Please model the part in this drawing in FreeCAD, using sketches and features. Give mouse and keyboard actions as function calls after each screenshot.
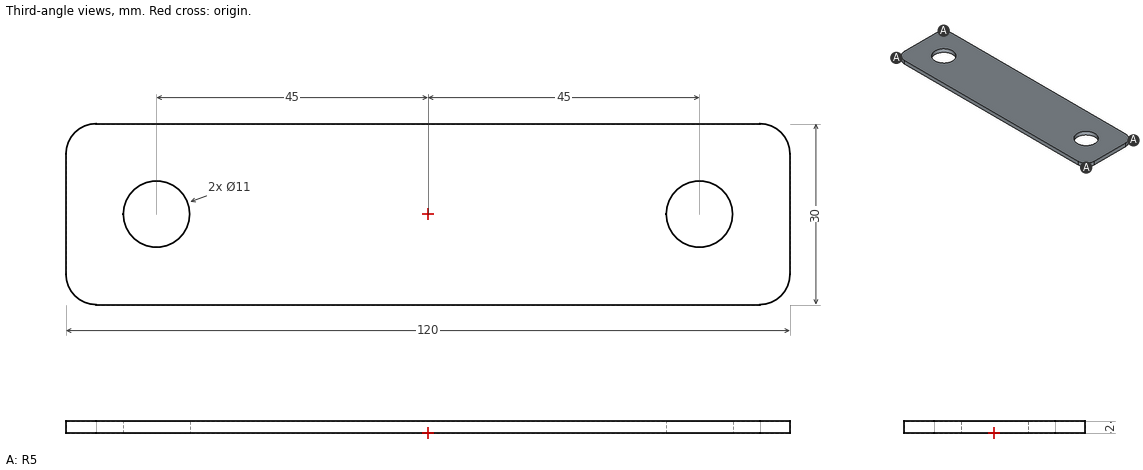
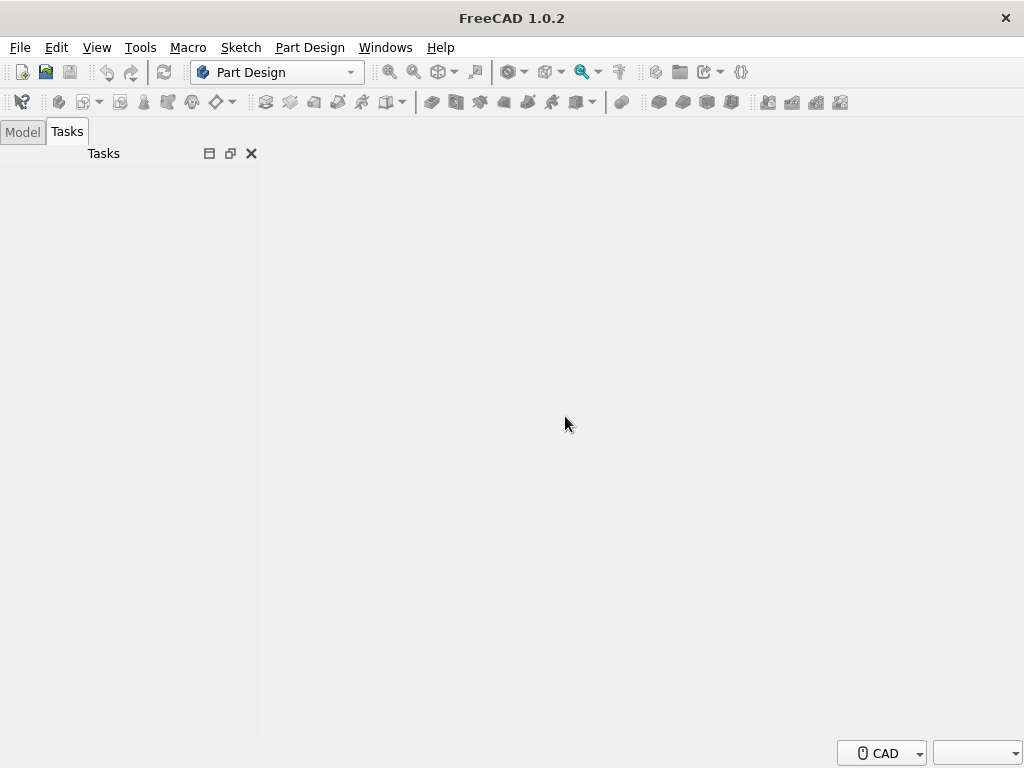
key(ctrl+n)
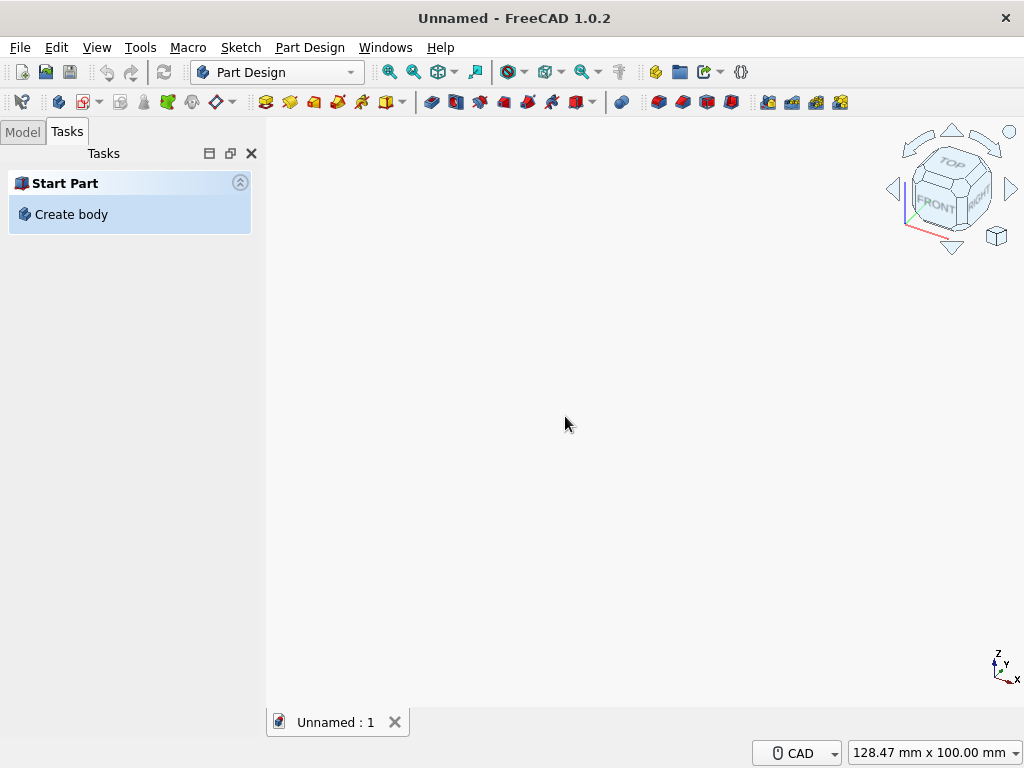
click(84, 102)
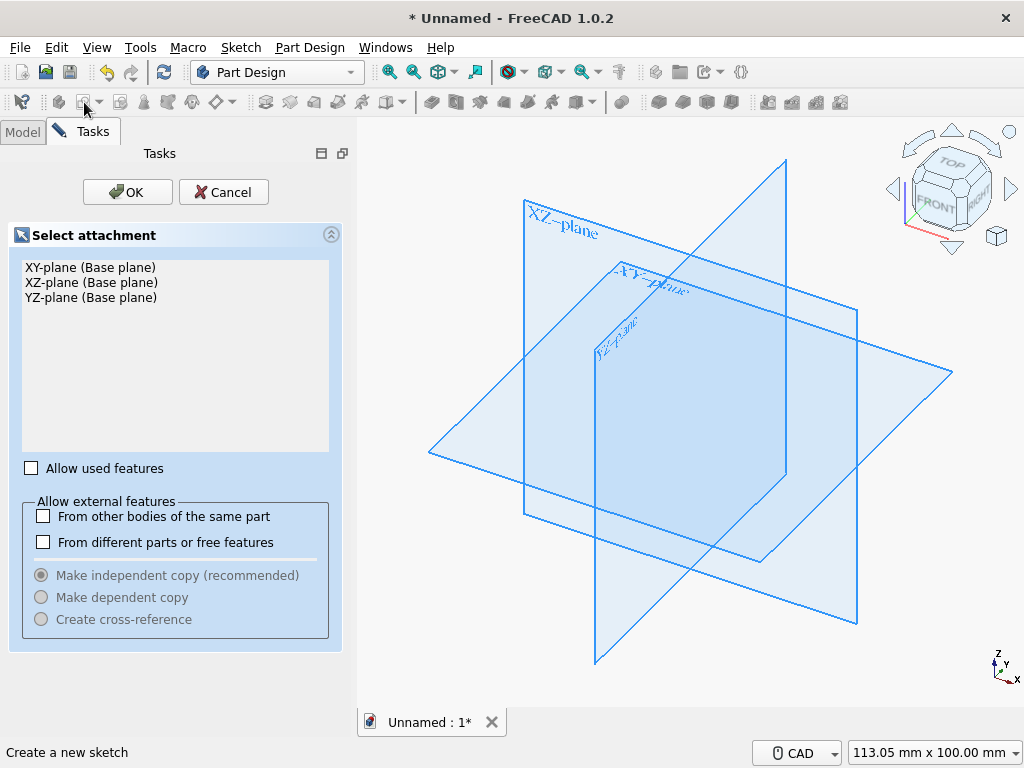
click(82, 268)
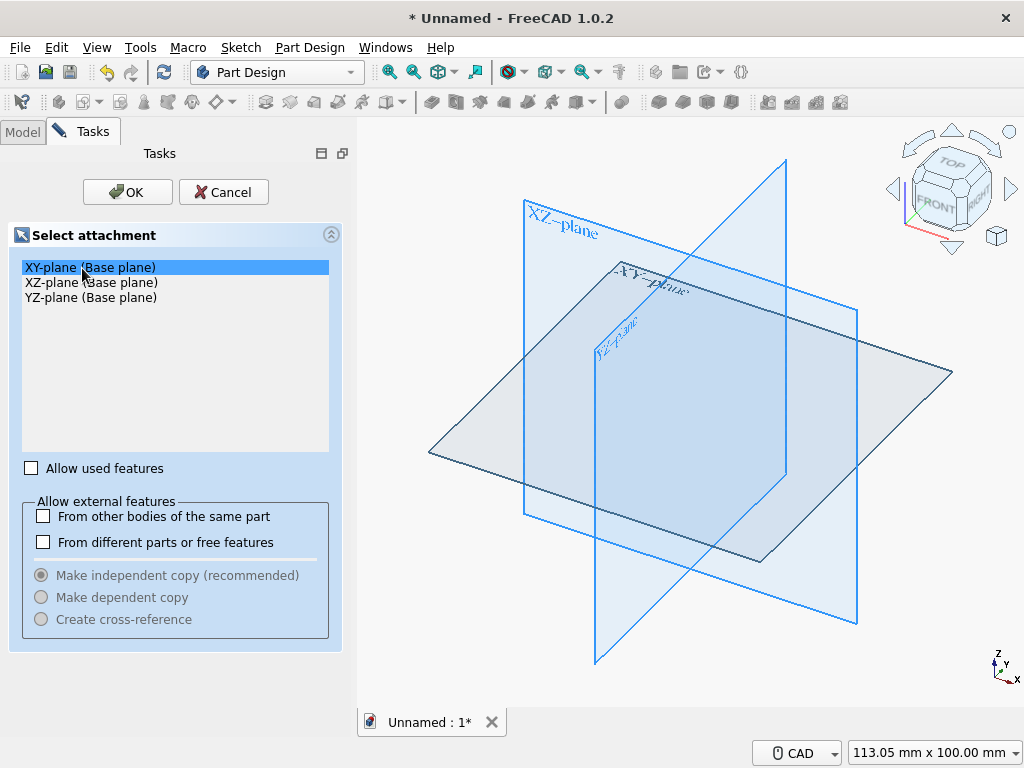
click(128, 192)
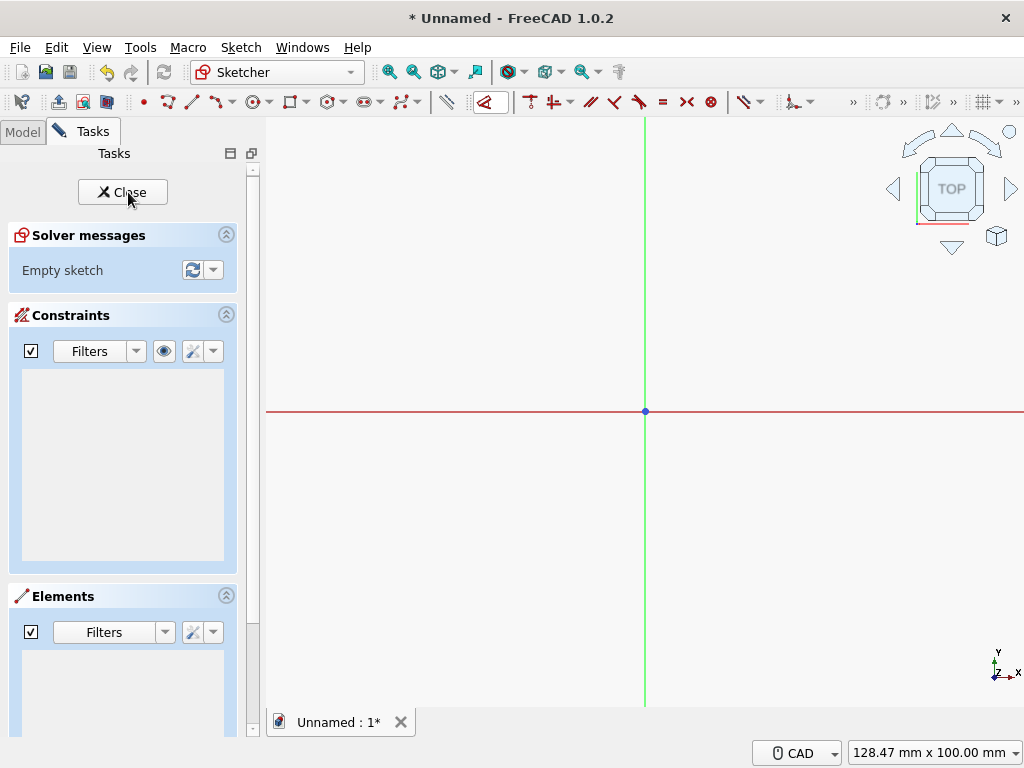
scroll(493, 412, down, 3)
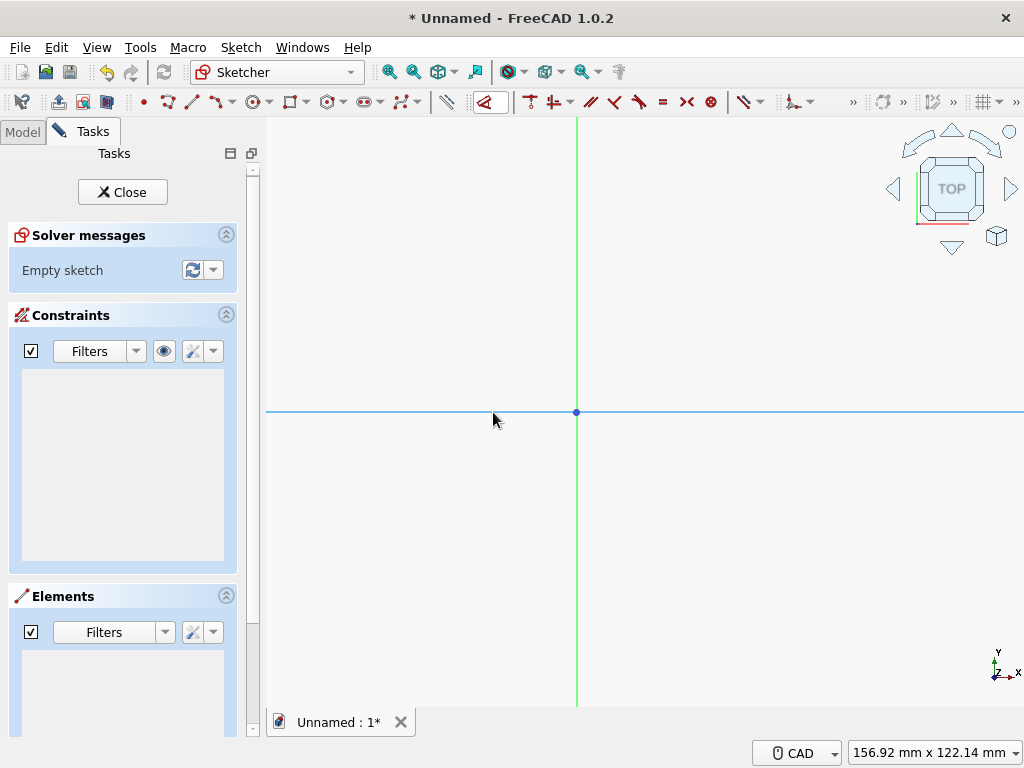
click(308, 102)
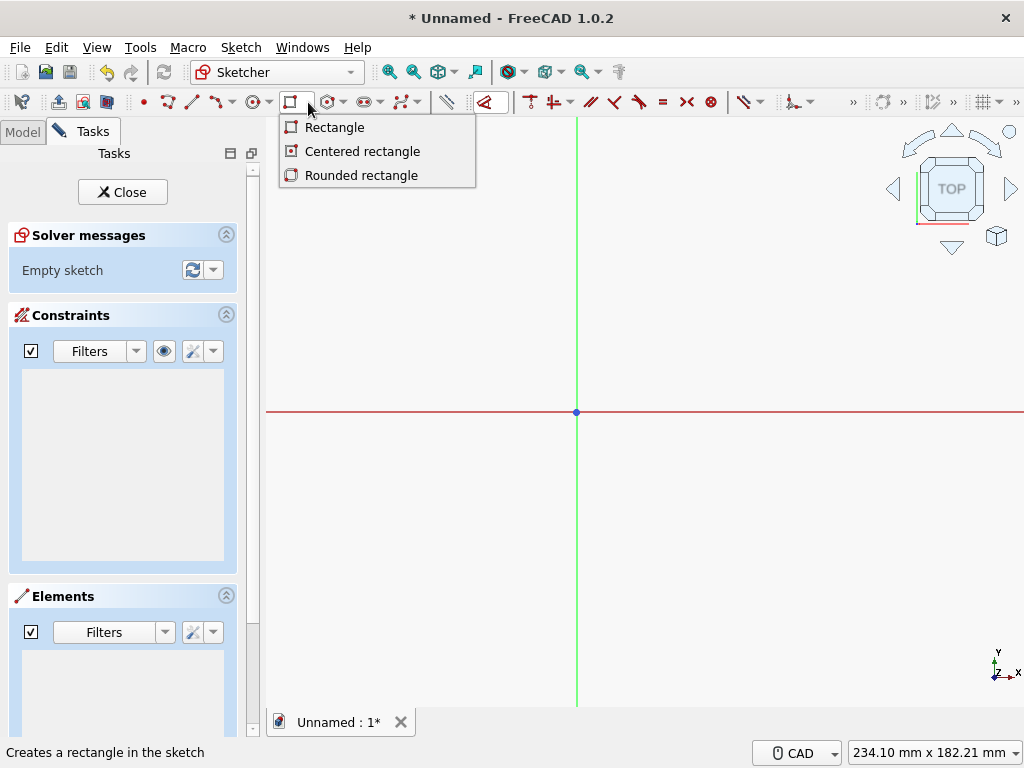
click(378, 151)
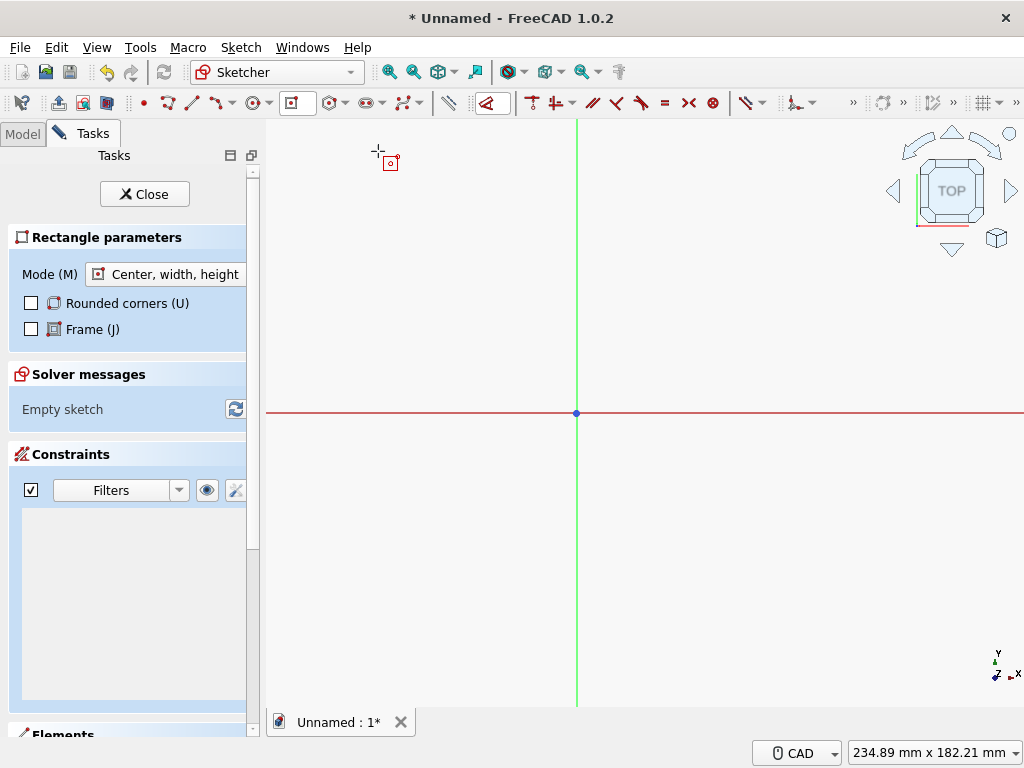
click(577, 413)
click(770, 365)
key(Escape)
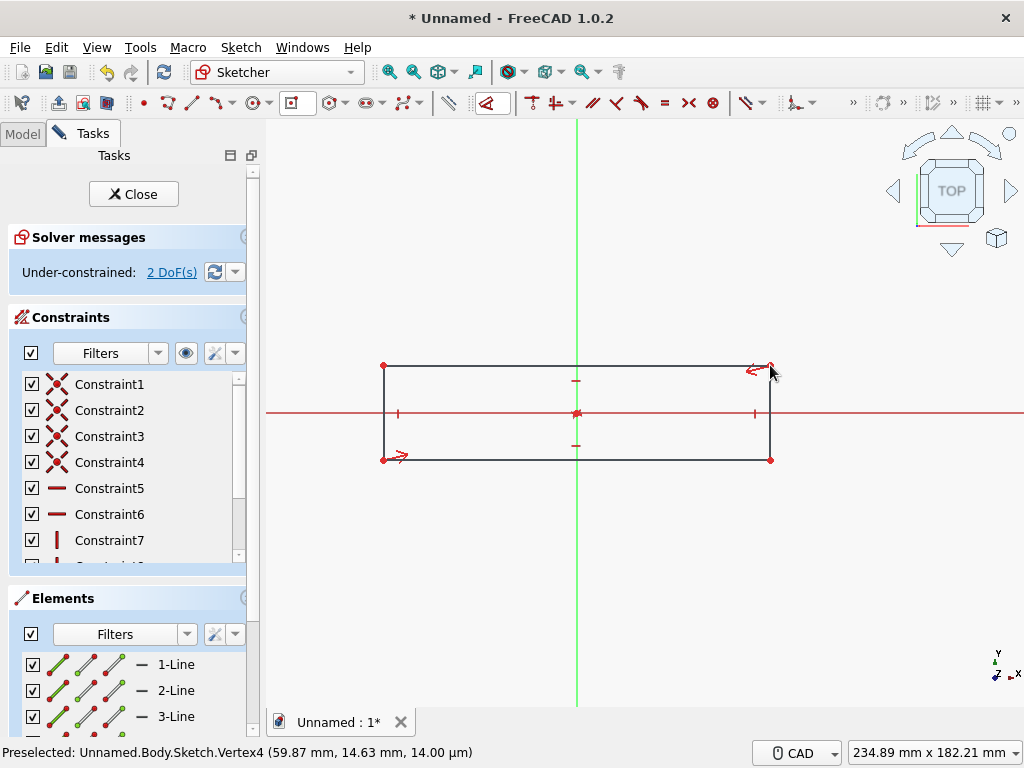
key(d)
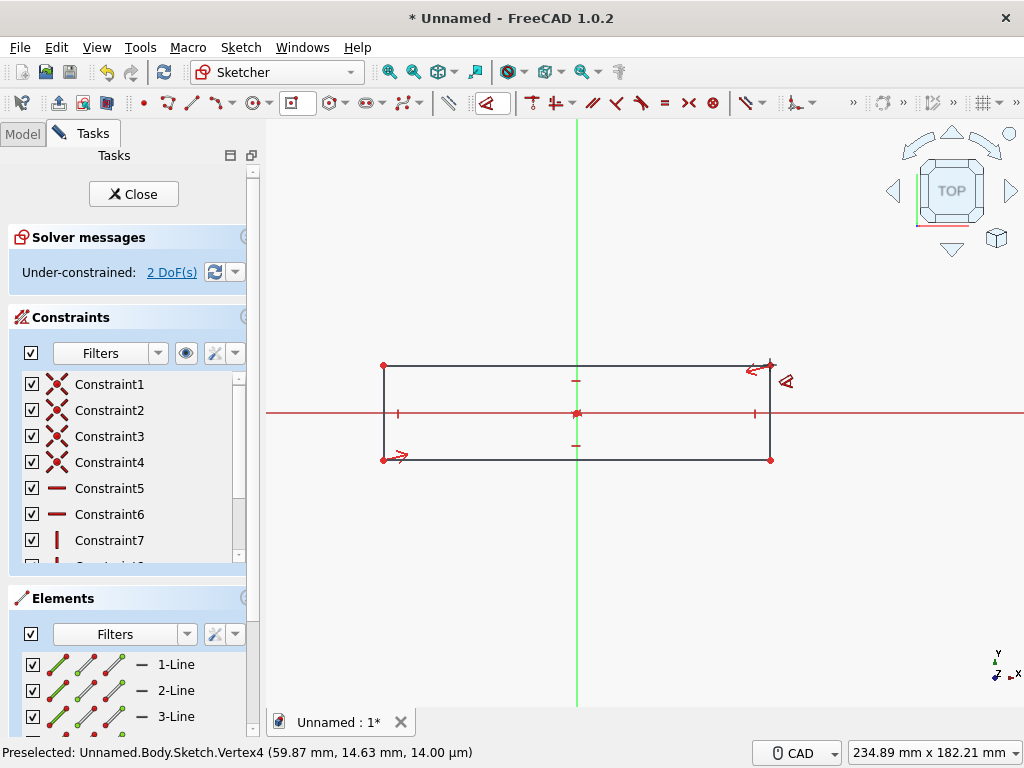
click(770, 432)
click(804, 392)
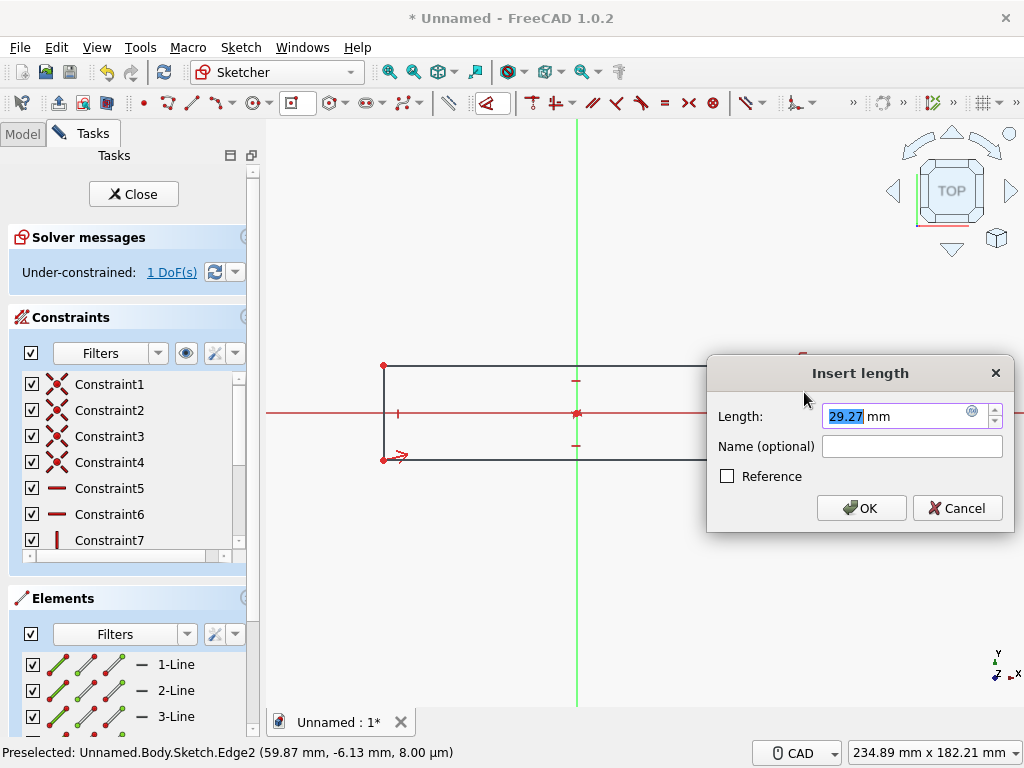
text(30)
key(Return)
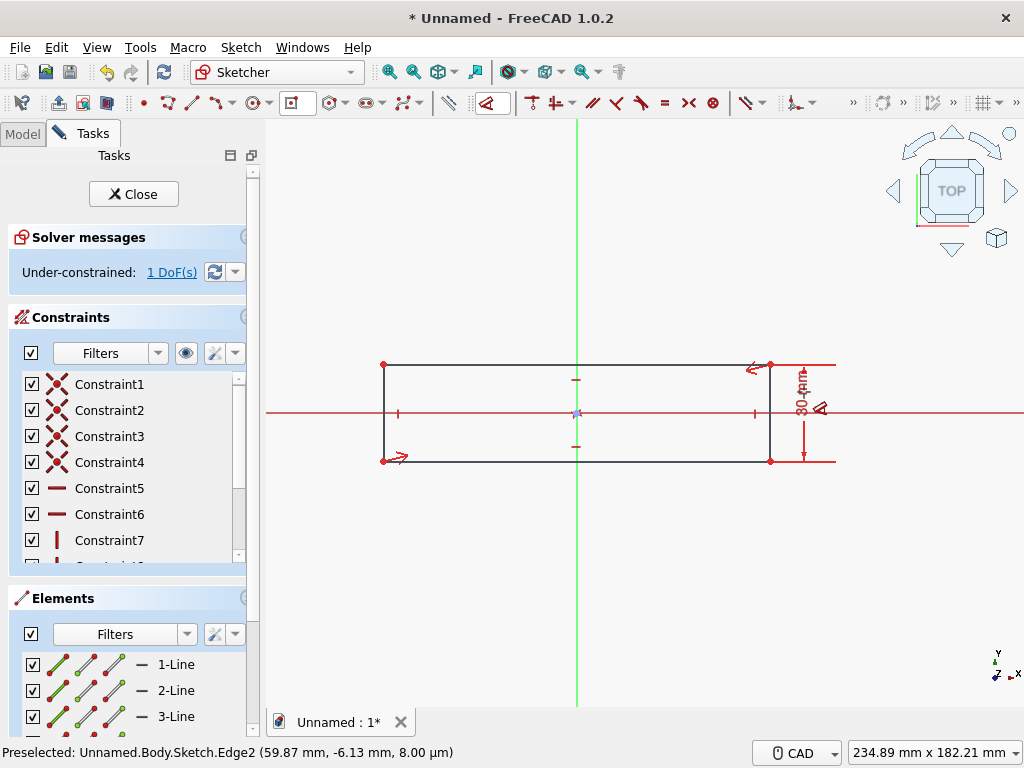
click(500, 462)
click(488, 496)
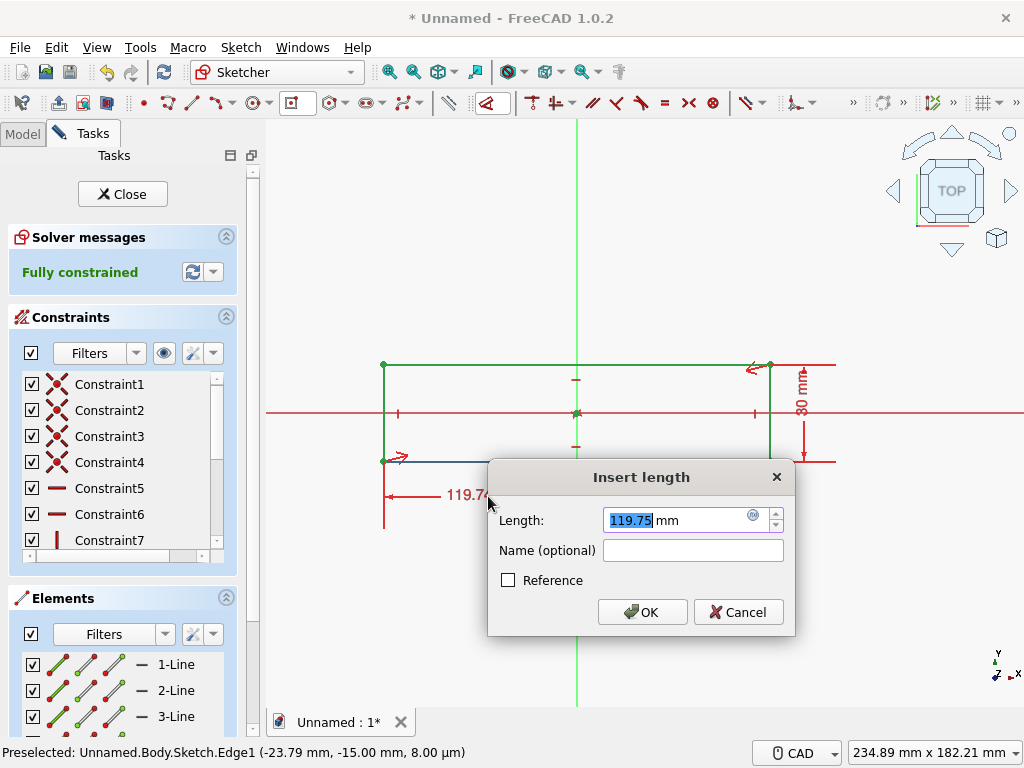
text(120)
key(Return)
key(Escape)